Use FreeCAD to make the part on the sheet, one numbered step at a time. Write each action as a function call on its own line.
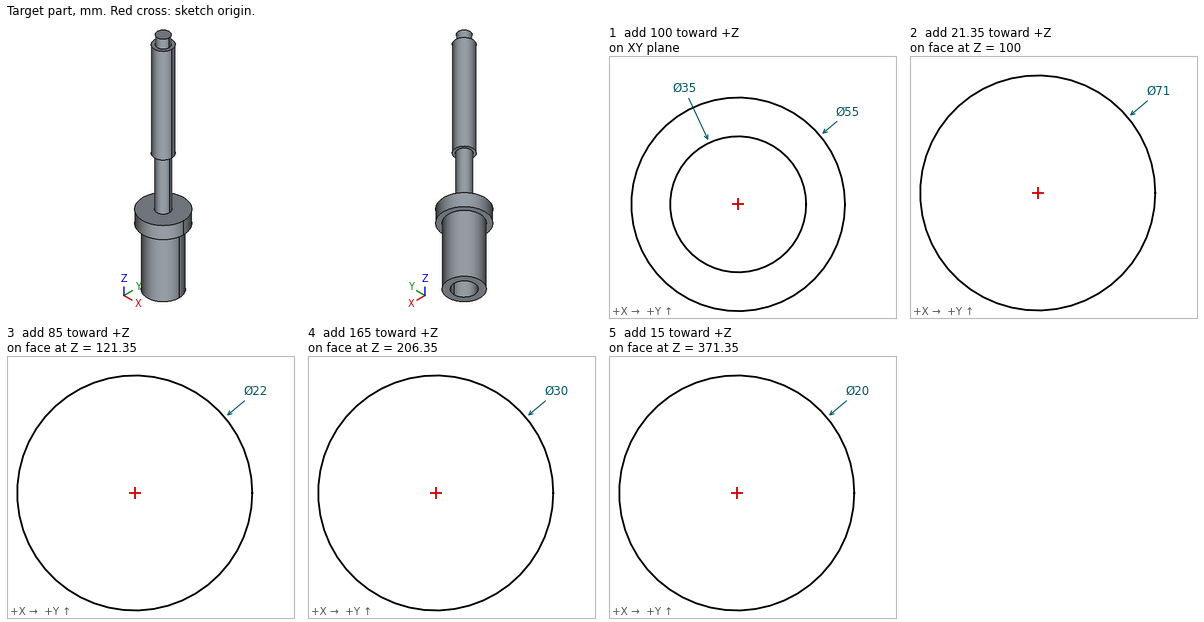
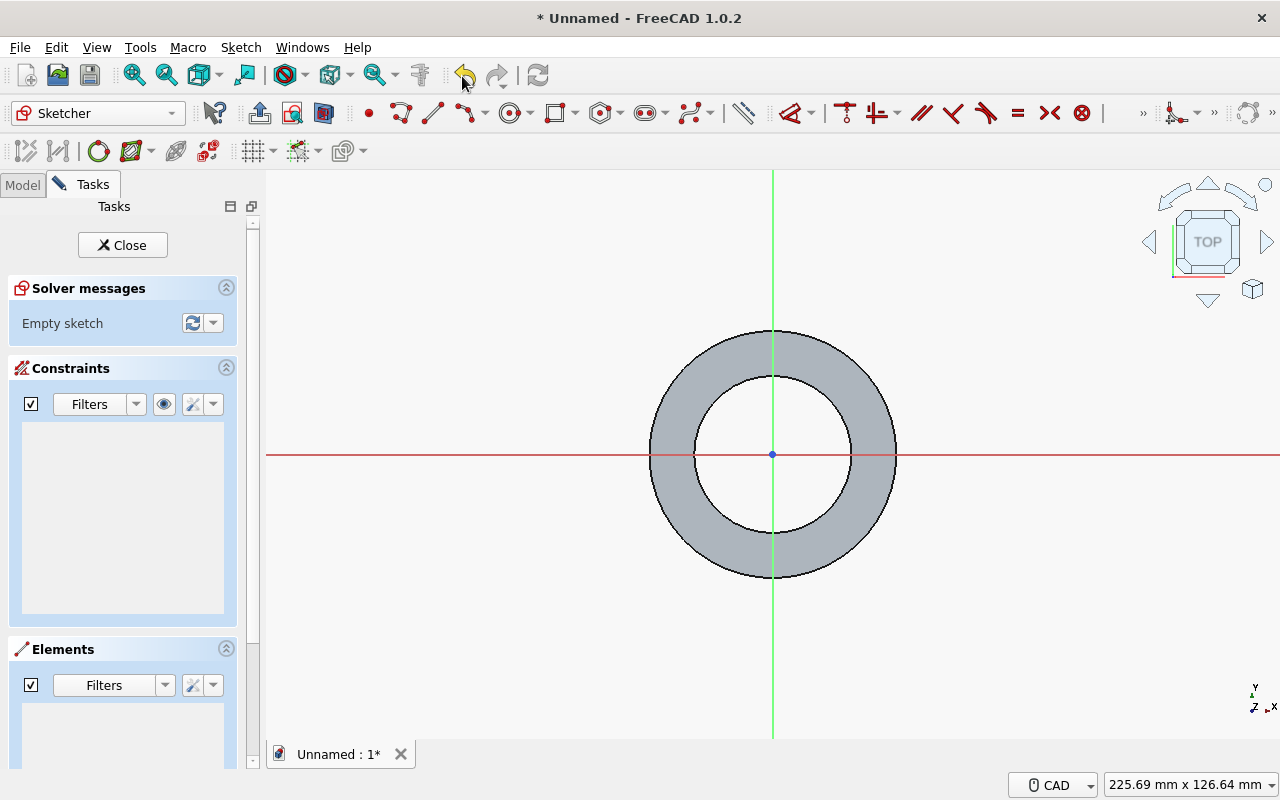
click(510, 114)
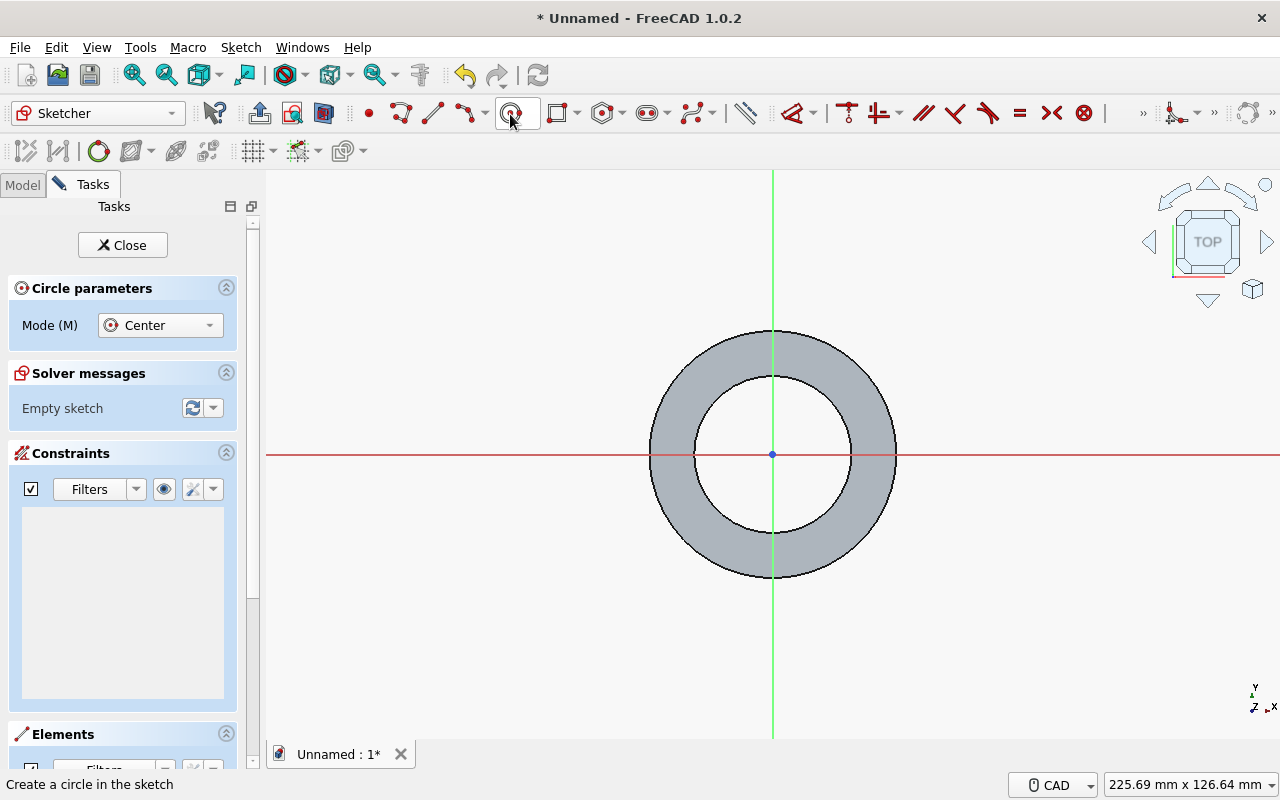
click(773, 454)
click(886, 342)
key(Escape)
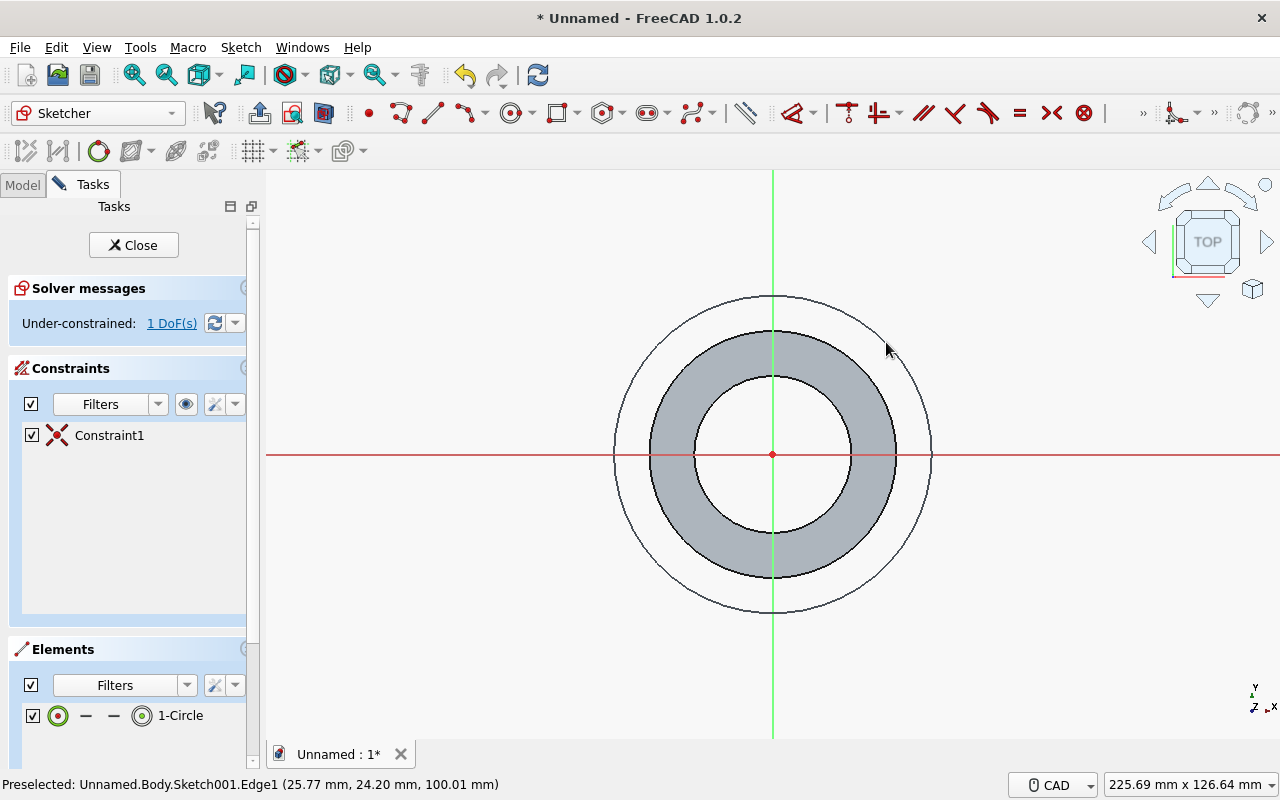
click(885, 342)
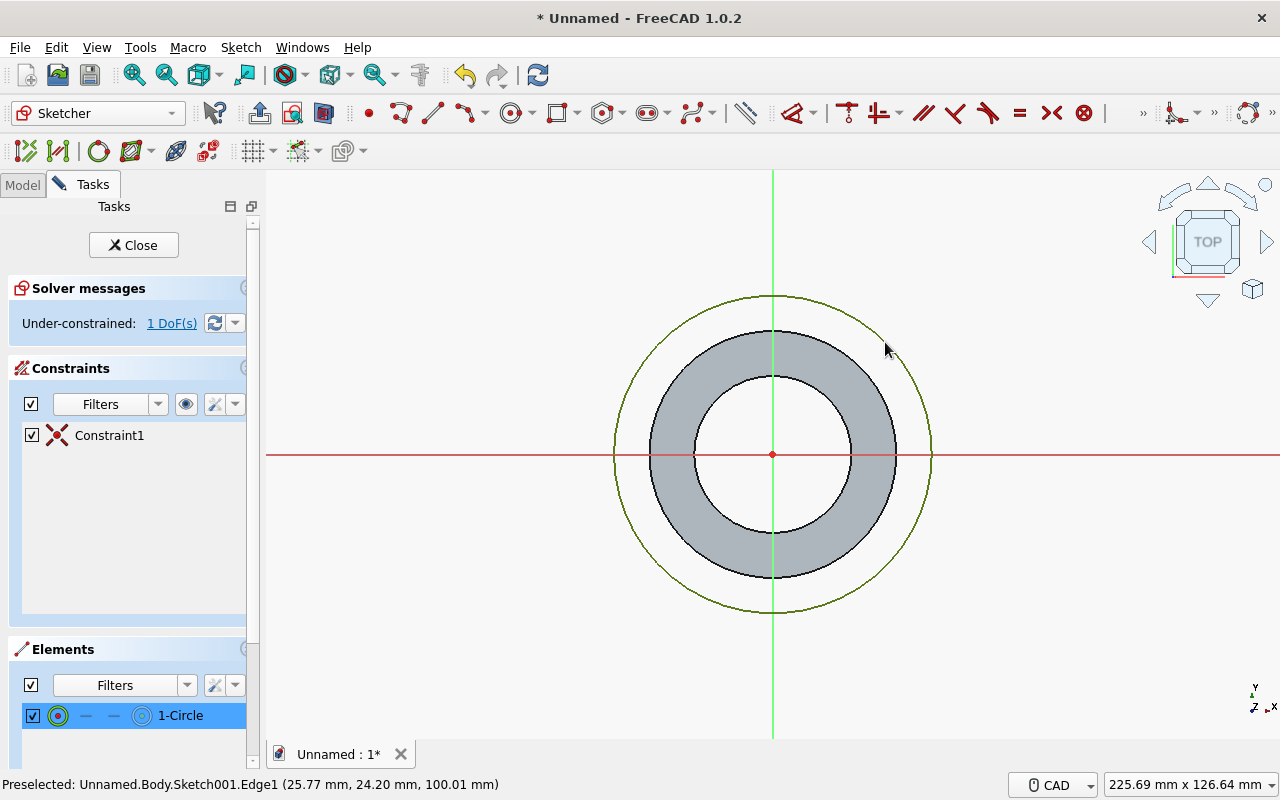
key(k)
key(o)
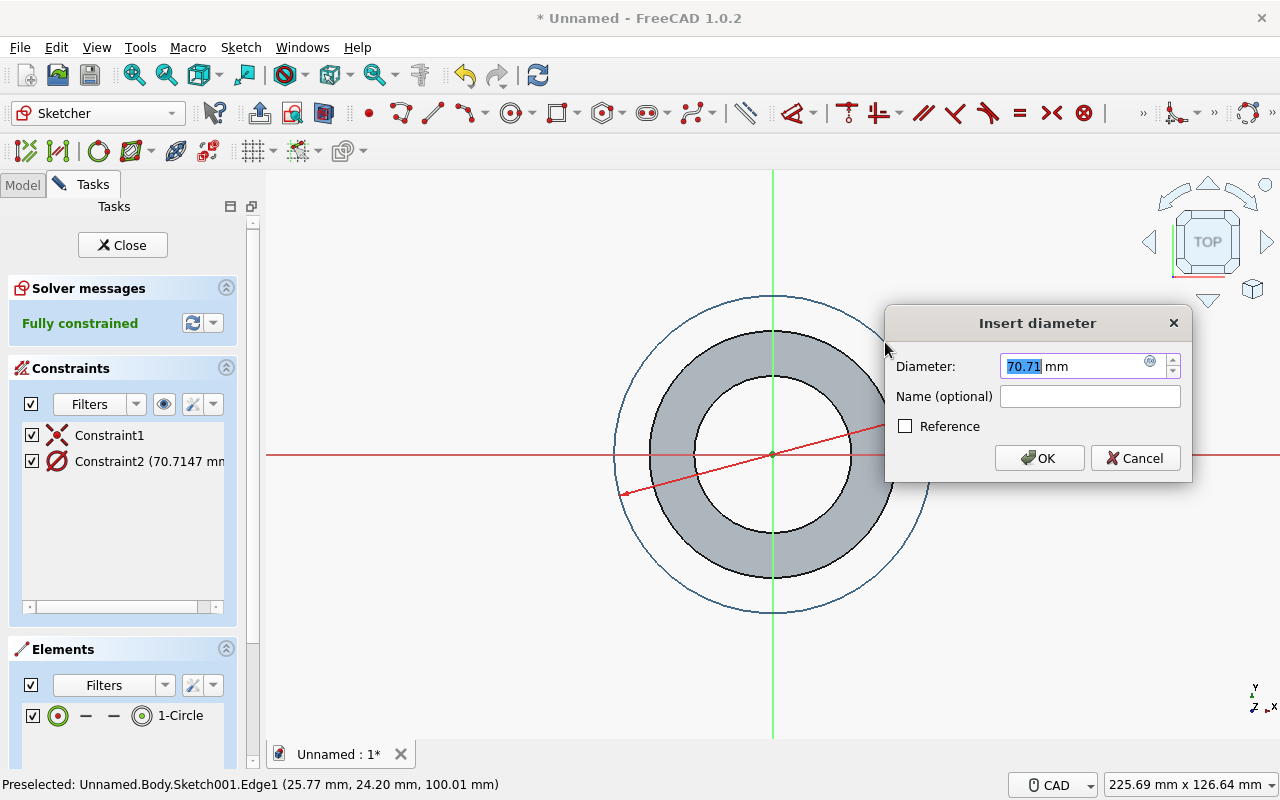
text(71)
key(Return)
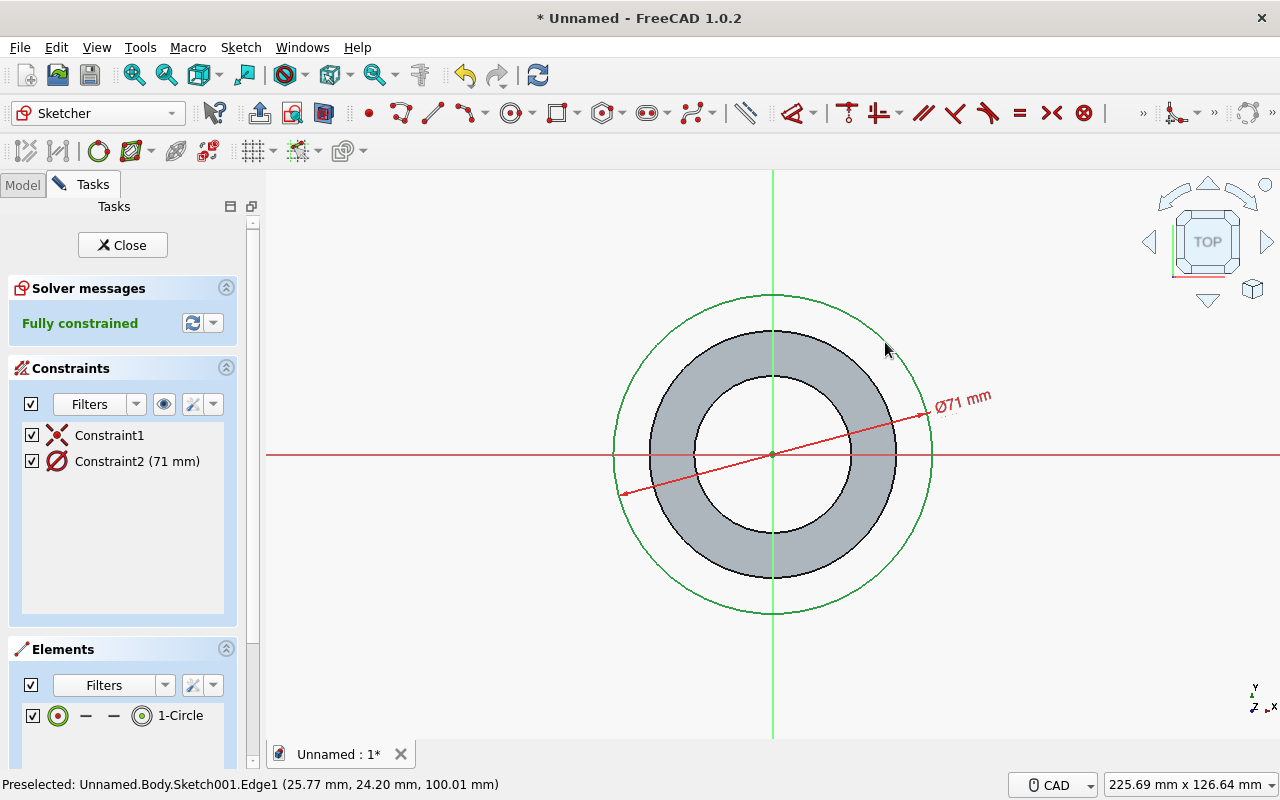
click(123, 245)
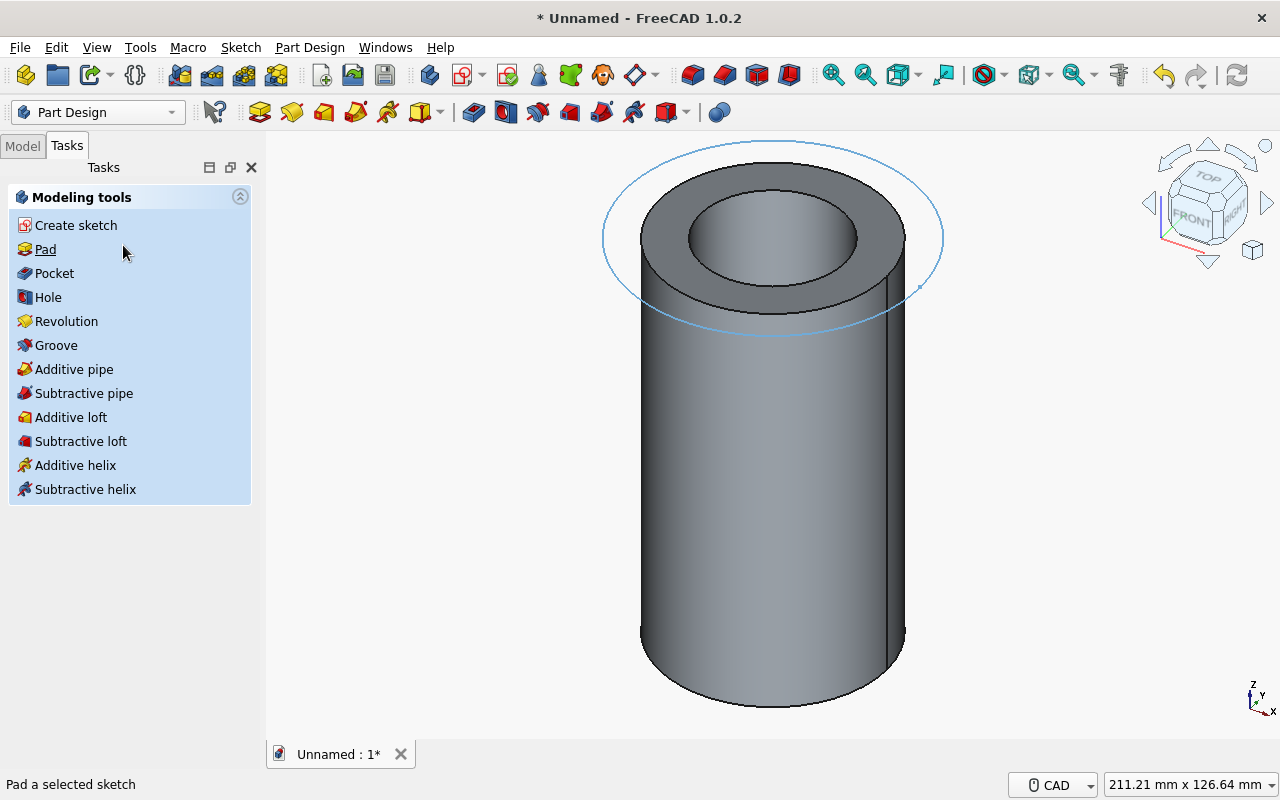
click(260, 112)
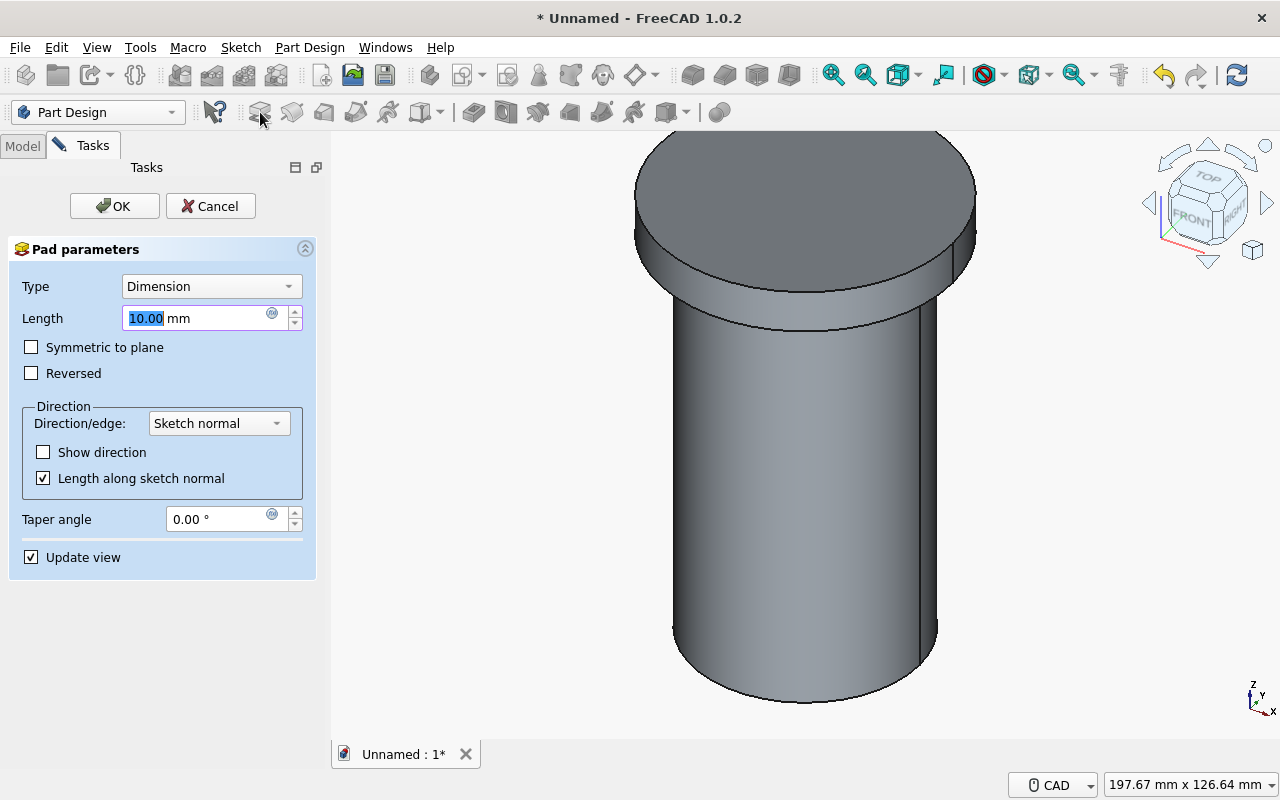
text(21.35)
key(Tab)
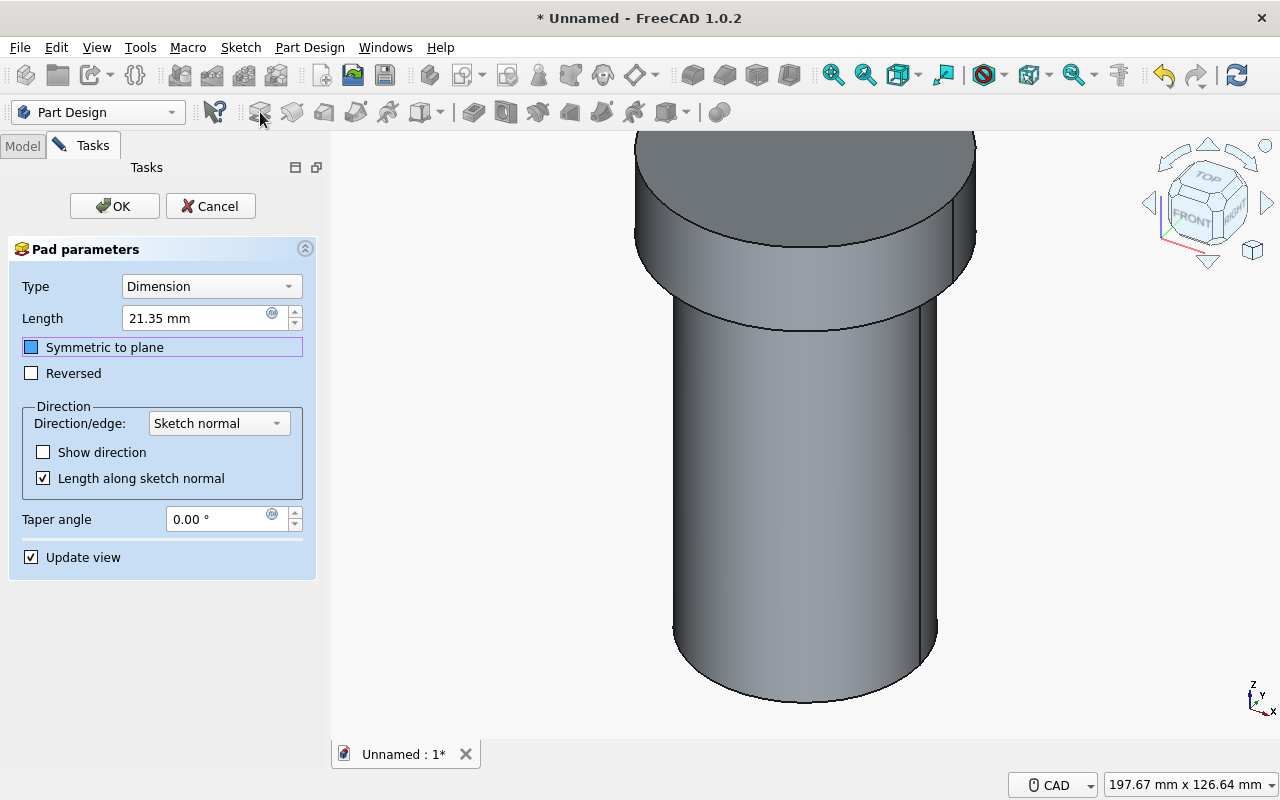
click(115, 206)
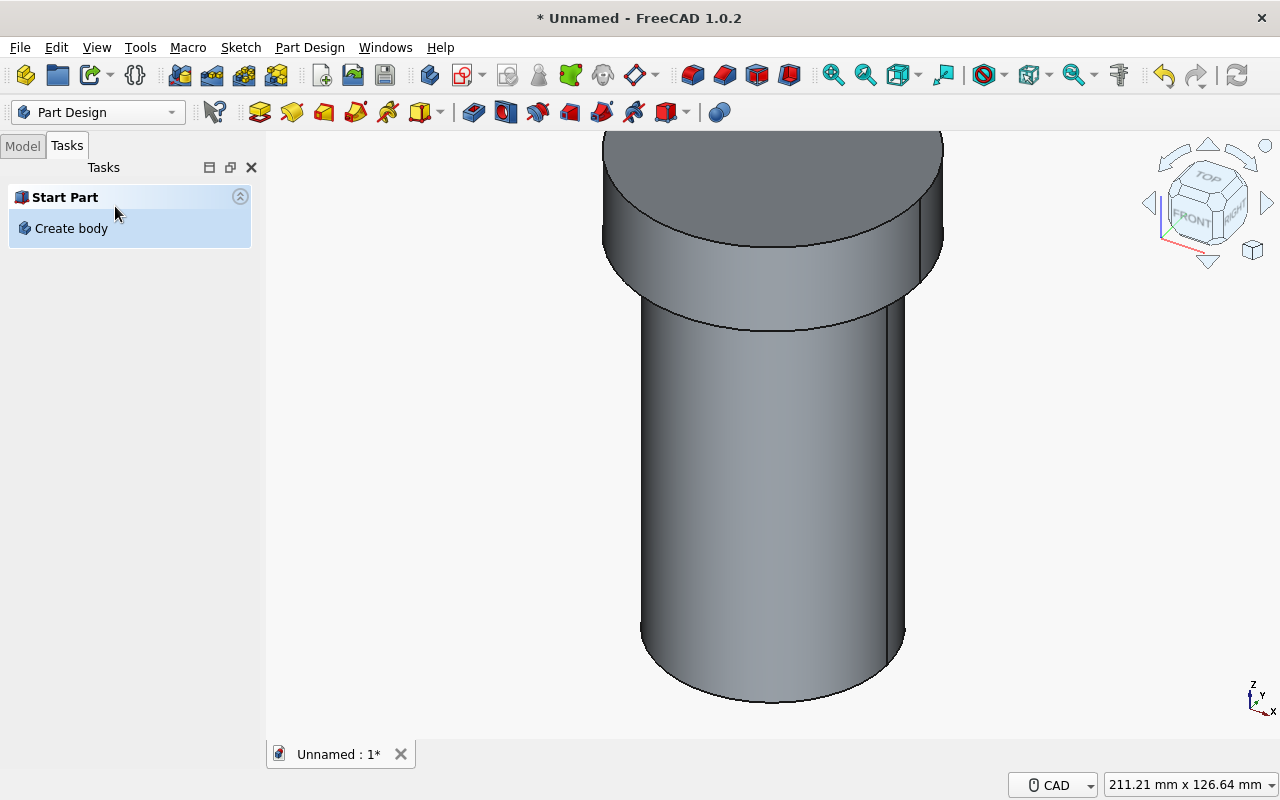
click(834, 76)